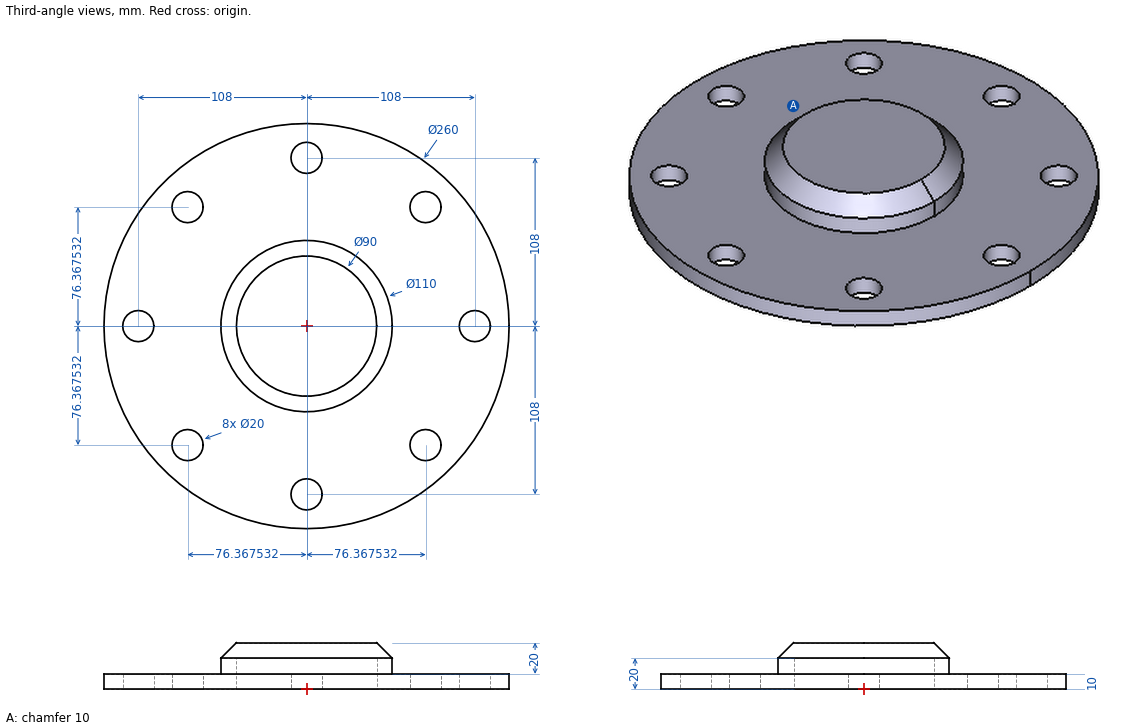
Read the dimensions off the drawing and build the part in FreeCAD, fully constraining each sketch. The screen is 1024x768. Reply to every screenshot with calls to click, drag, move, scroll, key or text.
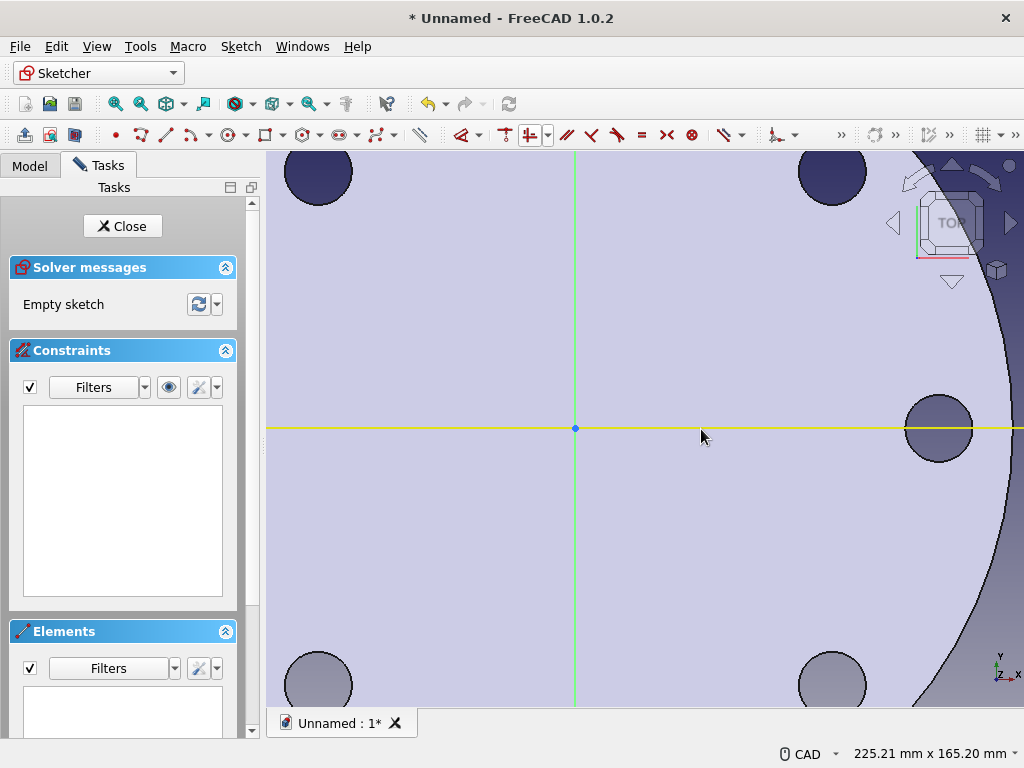
click(228, 136)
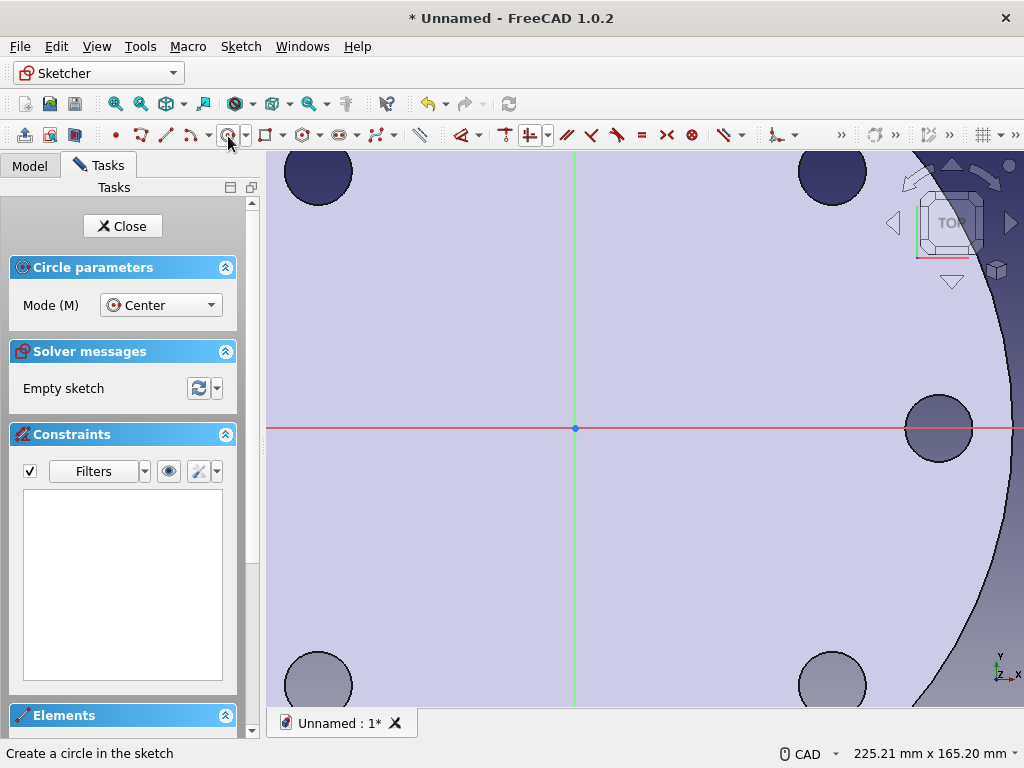
click(575, 428)
move(706, 297)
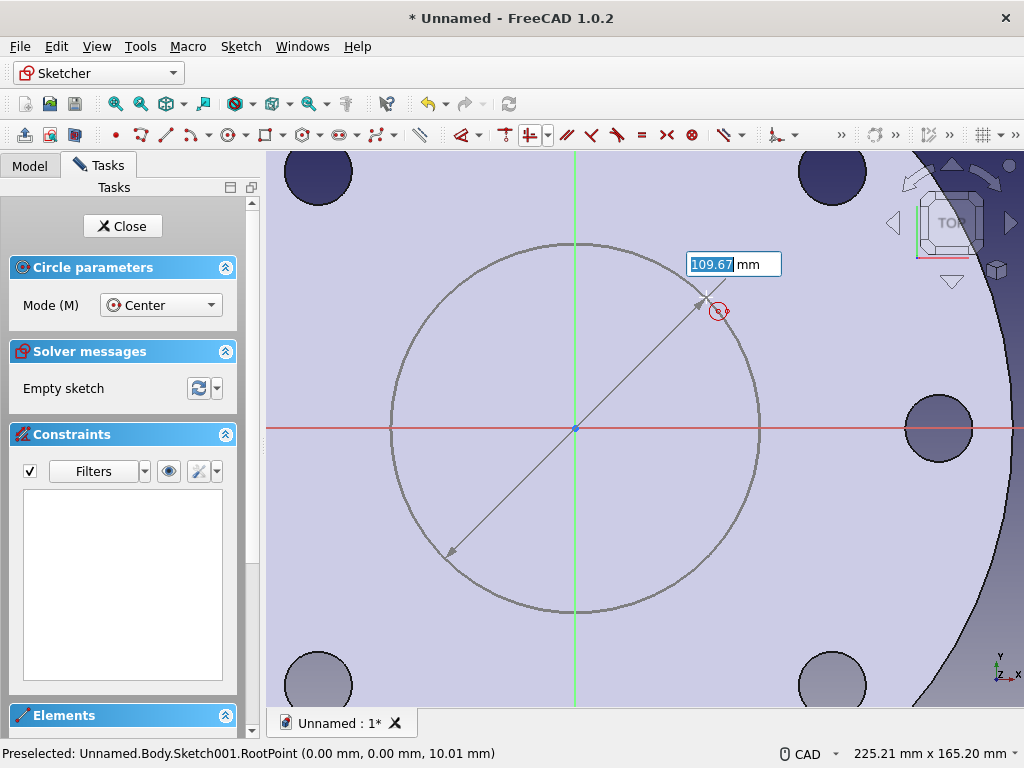
text(110)
key(Return)
key(Escape)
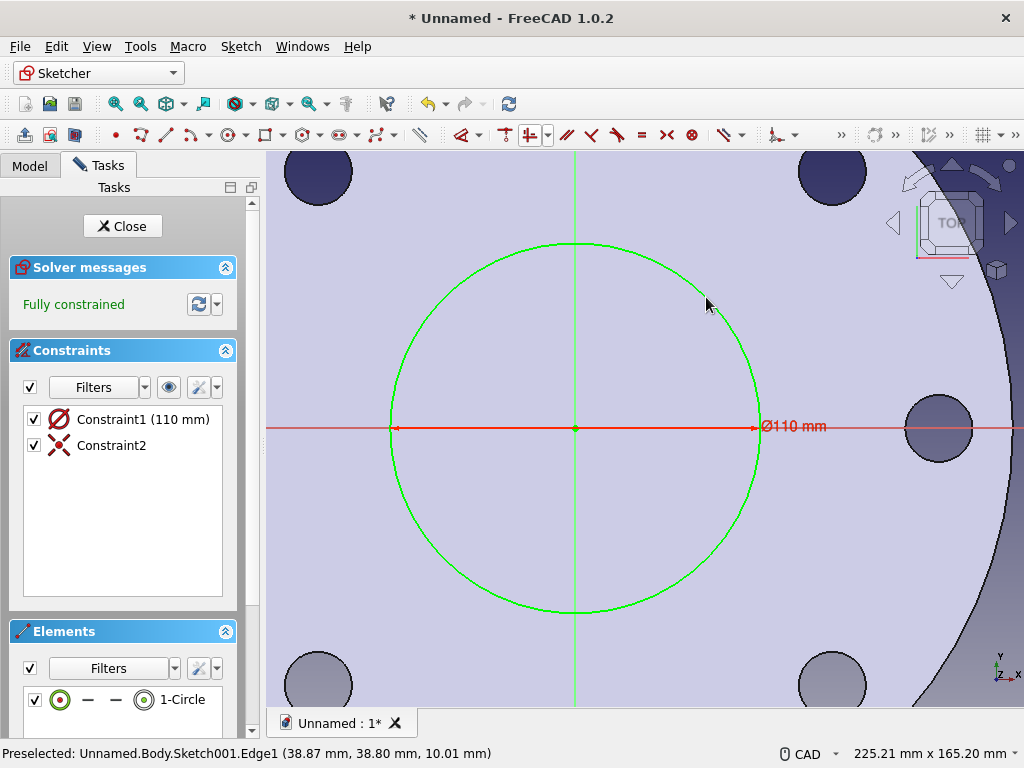
click(123, 226)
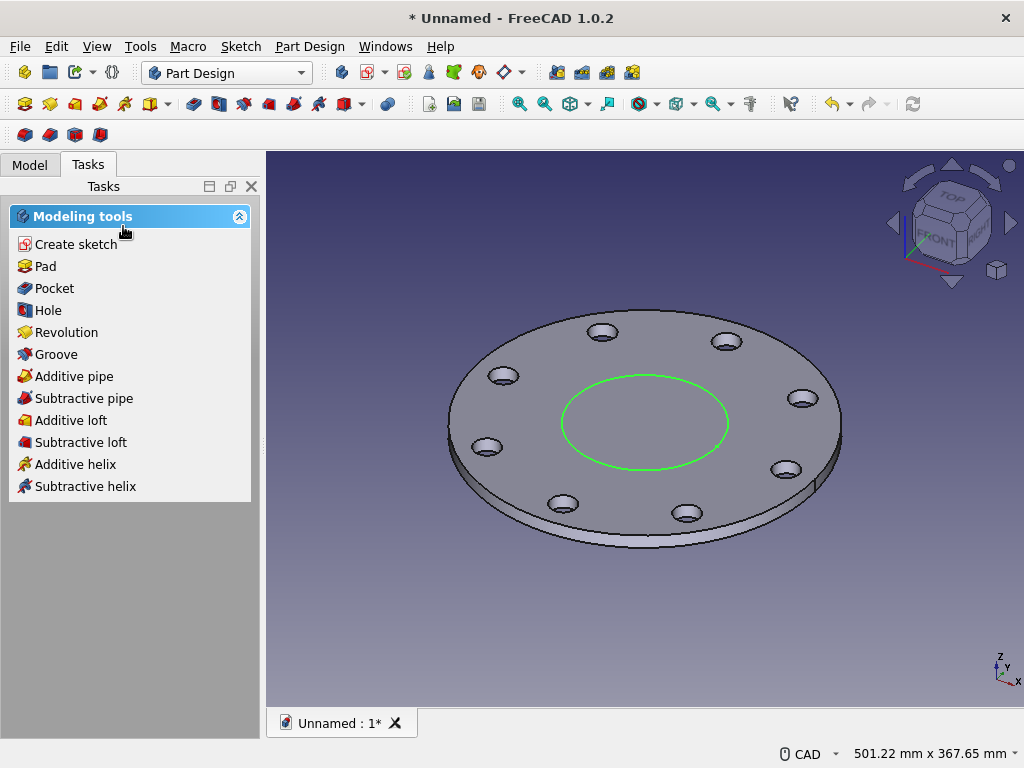
click(25, 104)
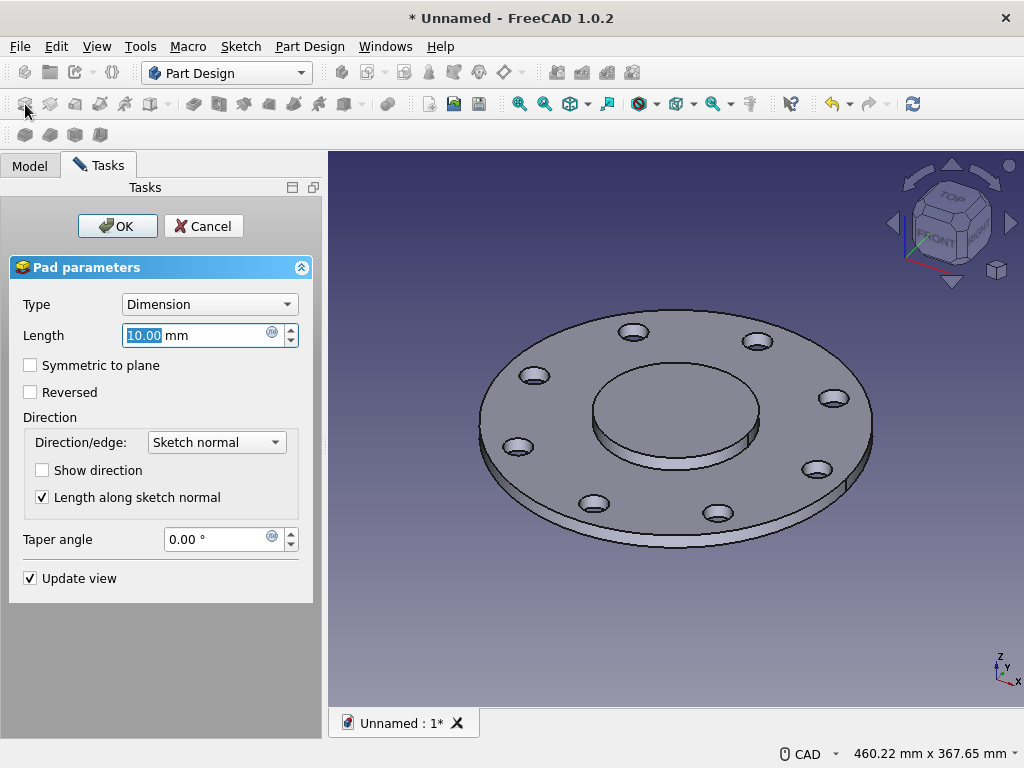
text(20)
key(Tab)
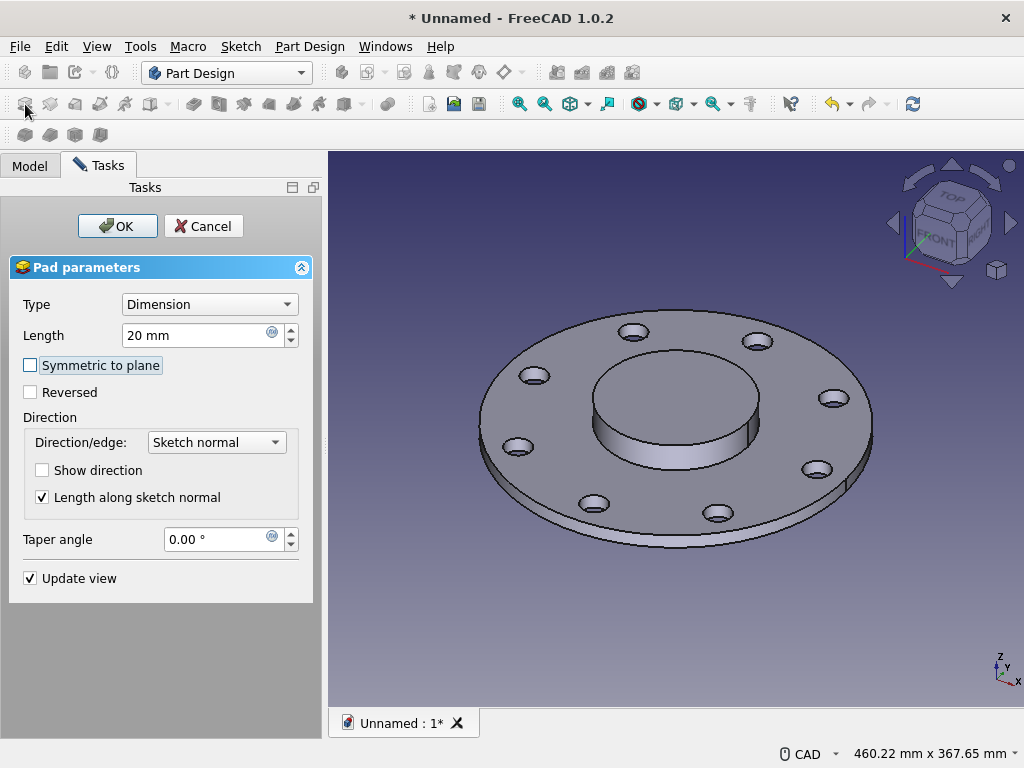
click(118, 226)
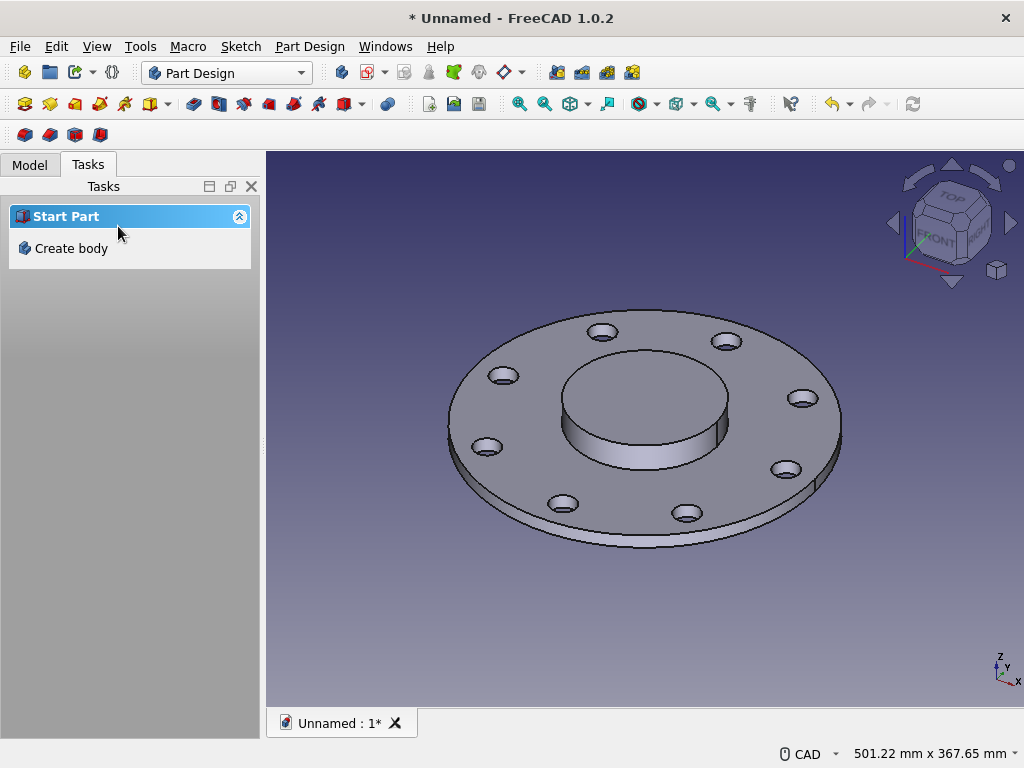
key(5)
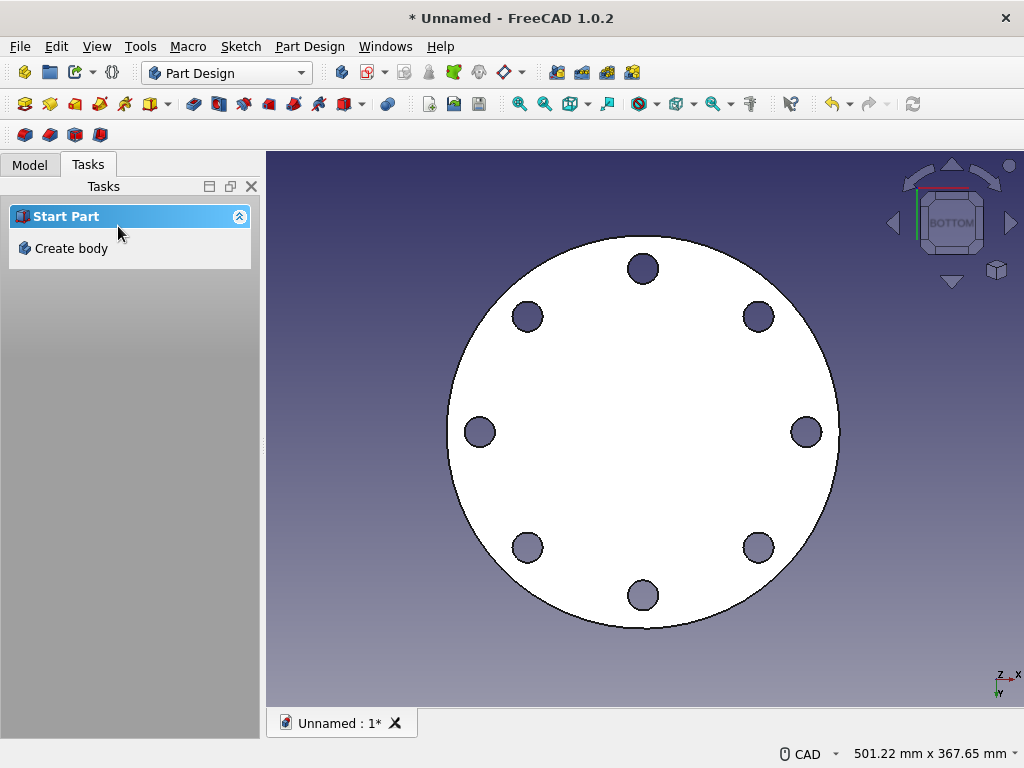
click(643, 431)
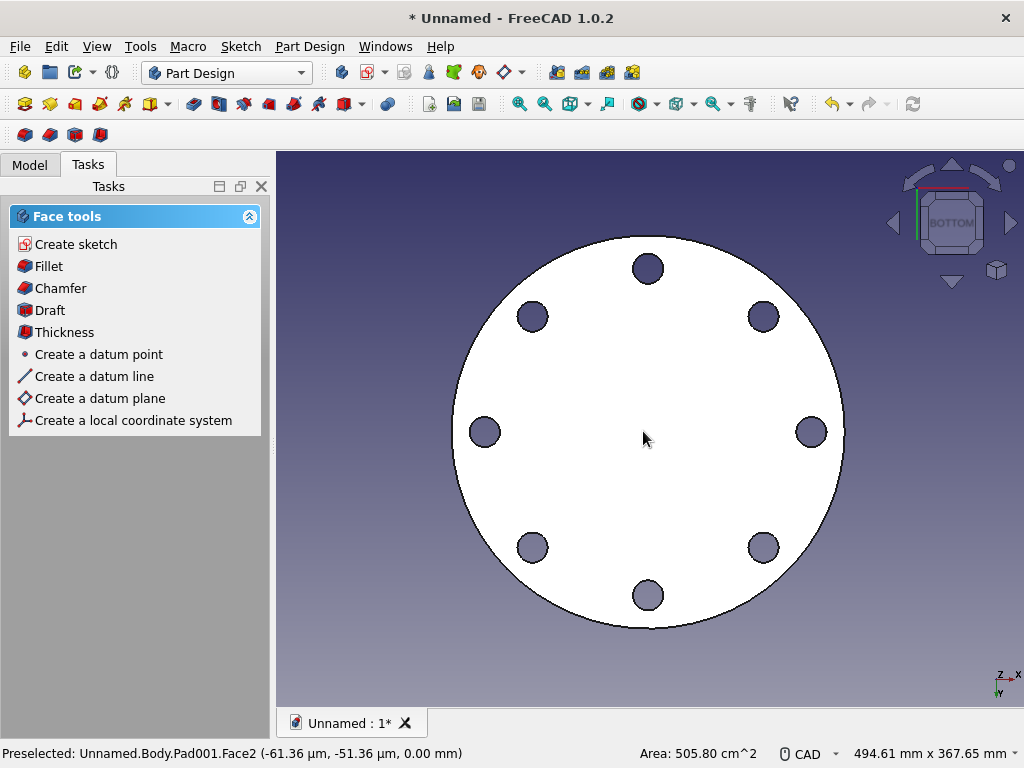
click(366, 72)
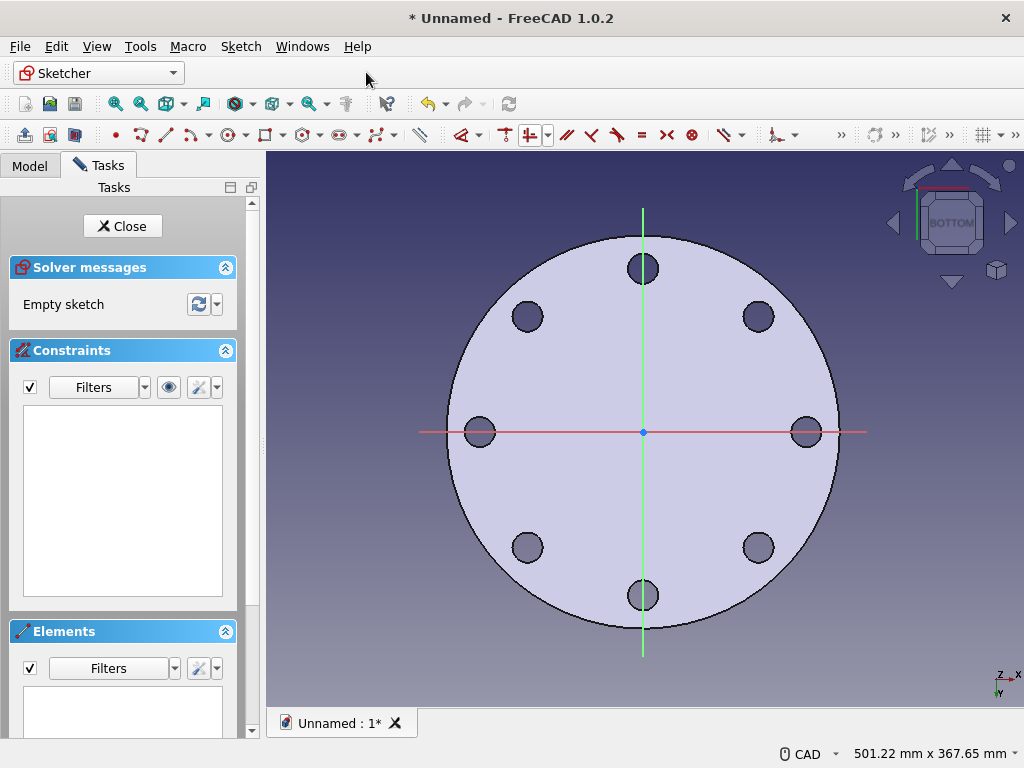
scroll(682, 434, up, 5)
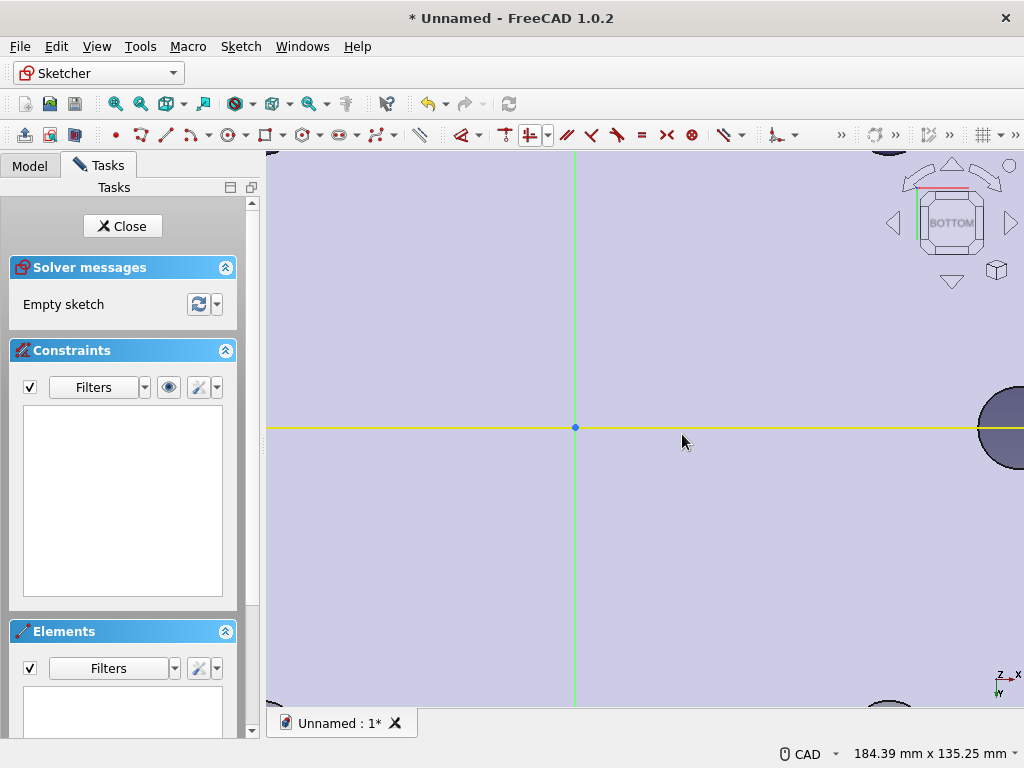
key(g)
key(c)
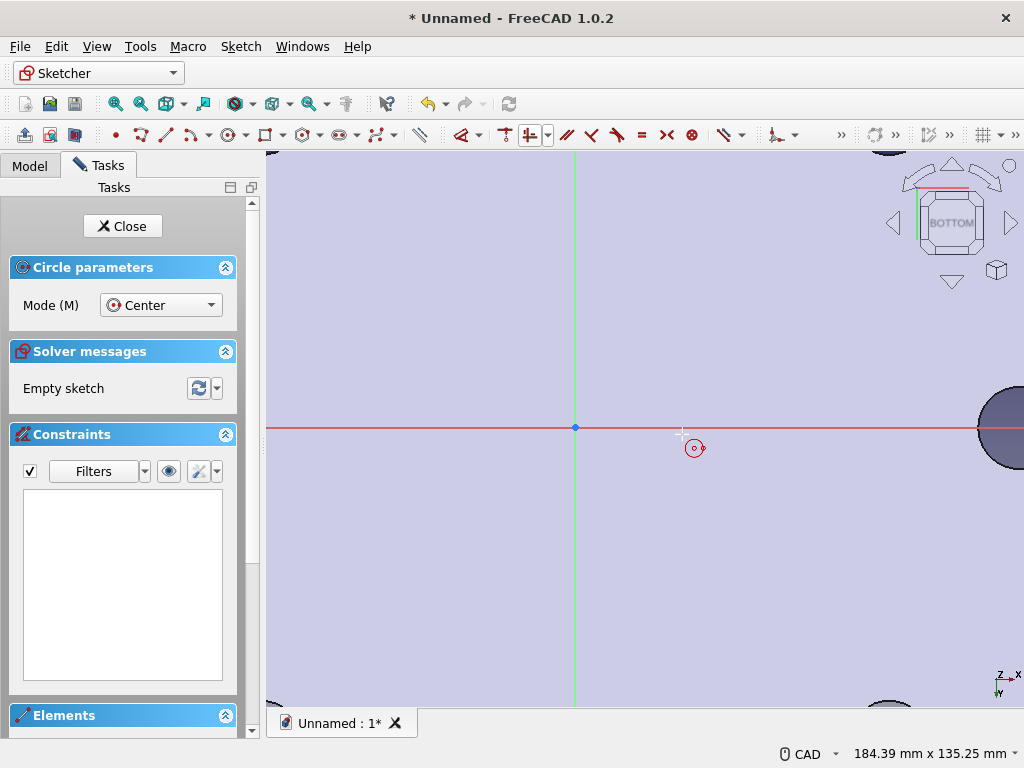
click(575, 428)
move(706, 297)